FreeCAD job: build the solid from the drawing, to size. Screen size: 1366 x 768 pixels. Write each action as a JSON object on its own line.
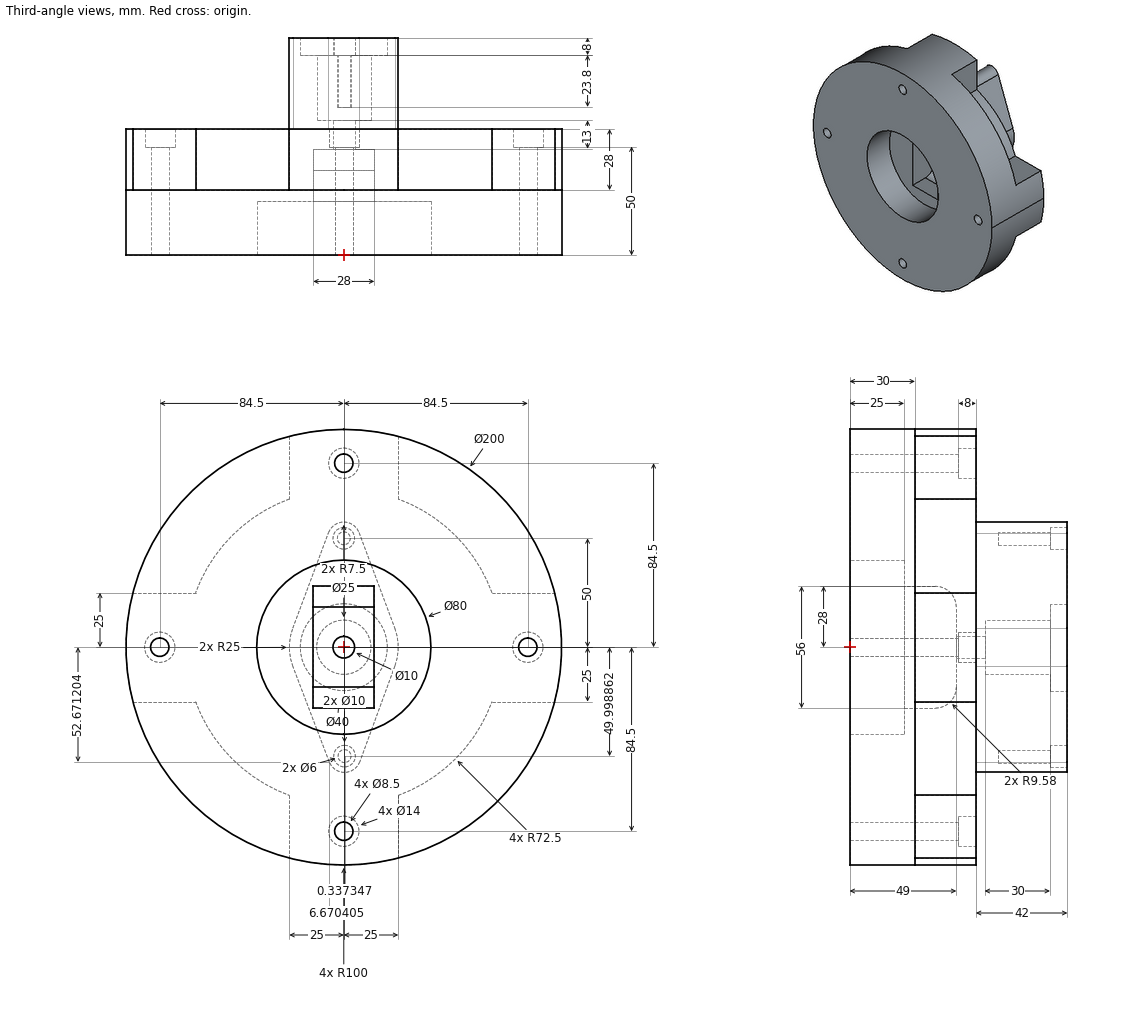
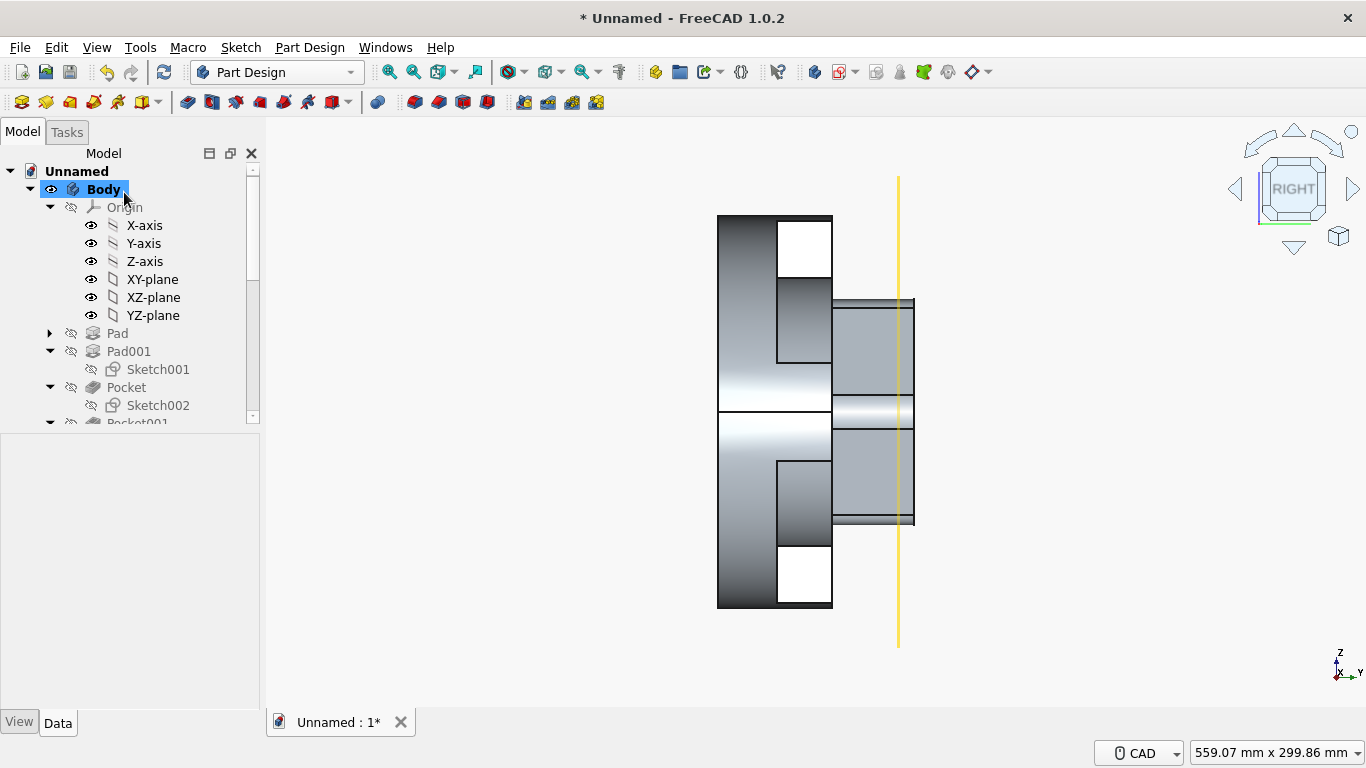
{"action": "scroll", "coordinate": [100, 293], "scroll_direction": "down", "scroll_amount": 3}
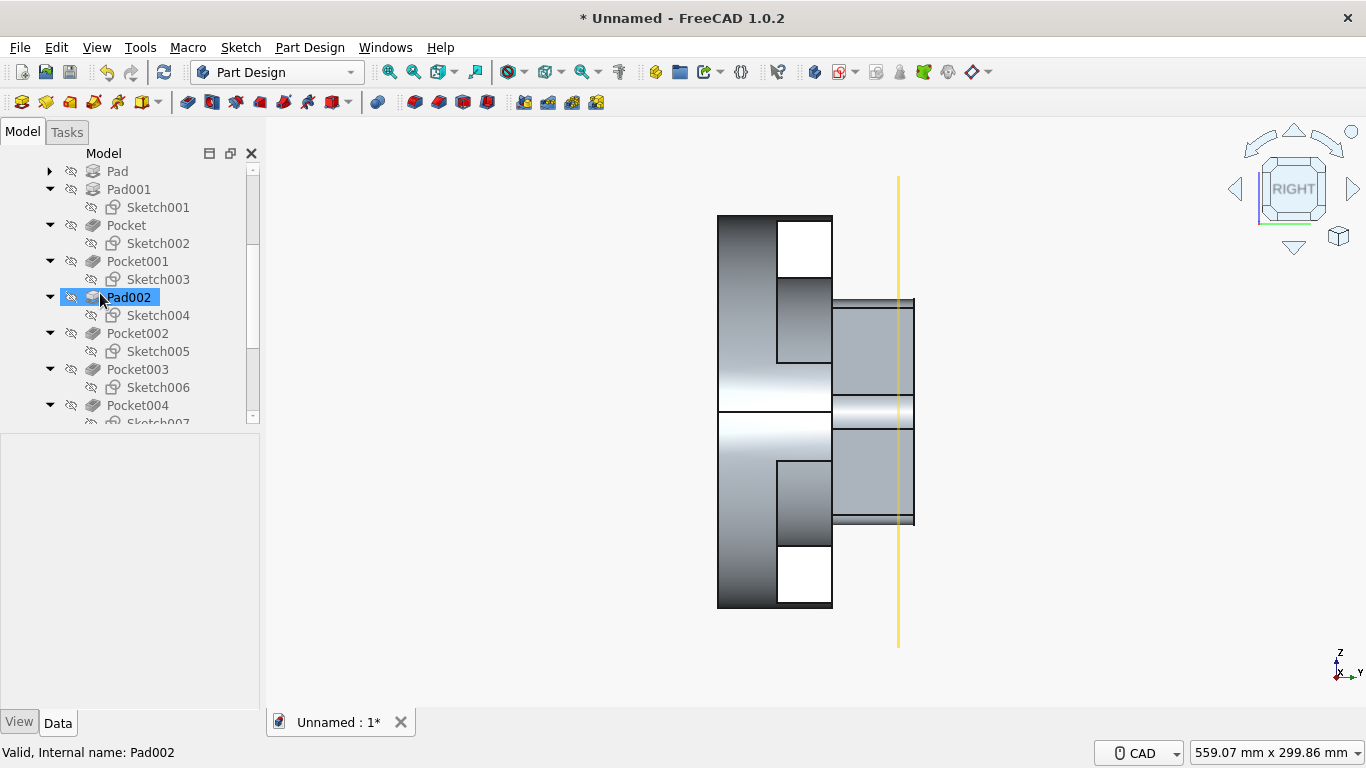
{"action": "scroll", "coordinate": [140, 293], "scroll_direction": "up", "scroll_amount": 15}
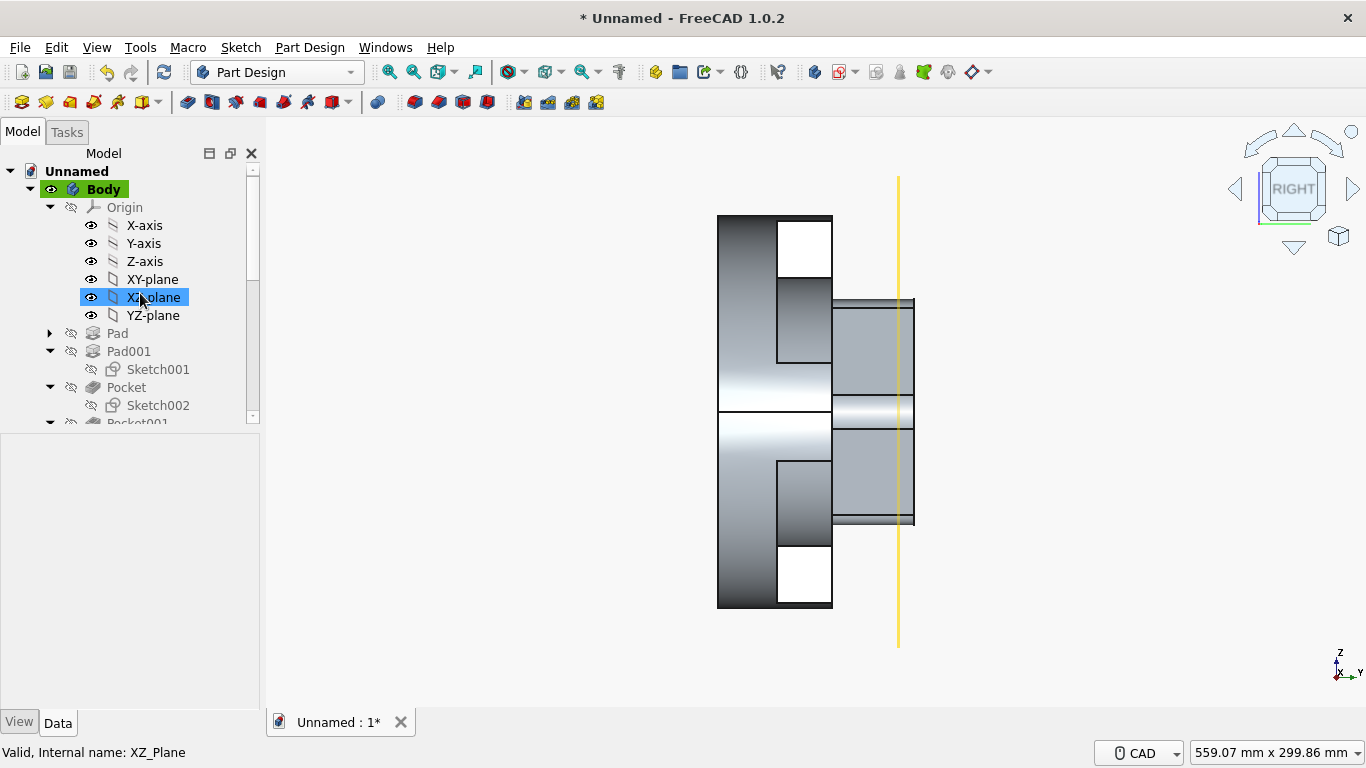
{"action": "scroll", "coordinate": [100, 293], "scroll_direction": "down", "scroll_amount": 6}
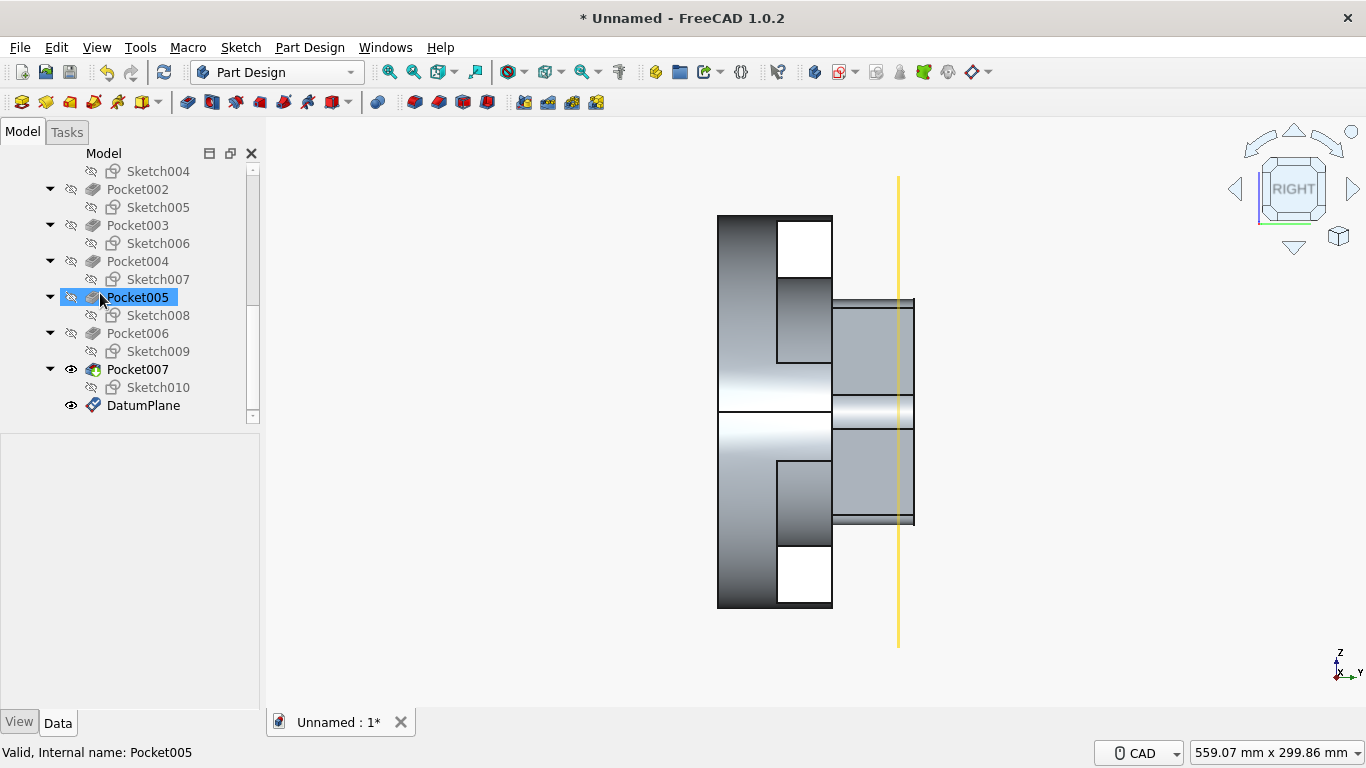
{"action": "left_click", "coordinate": [116, 405]}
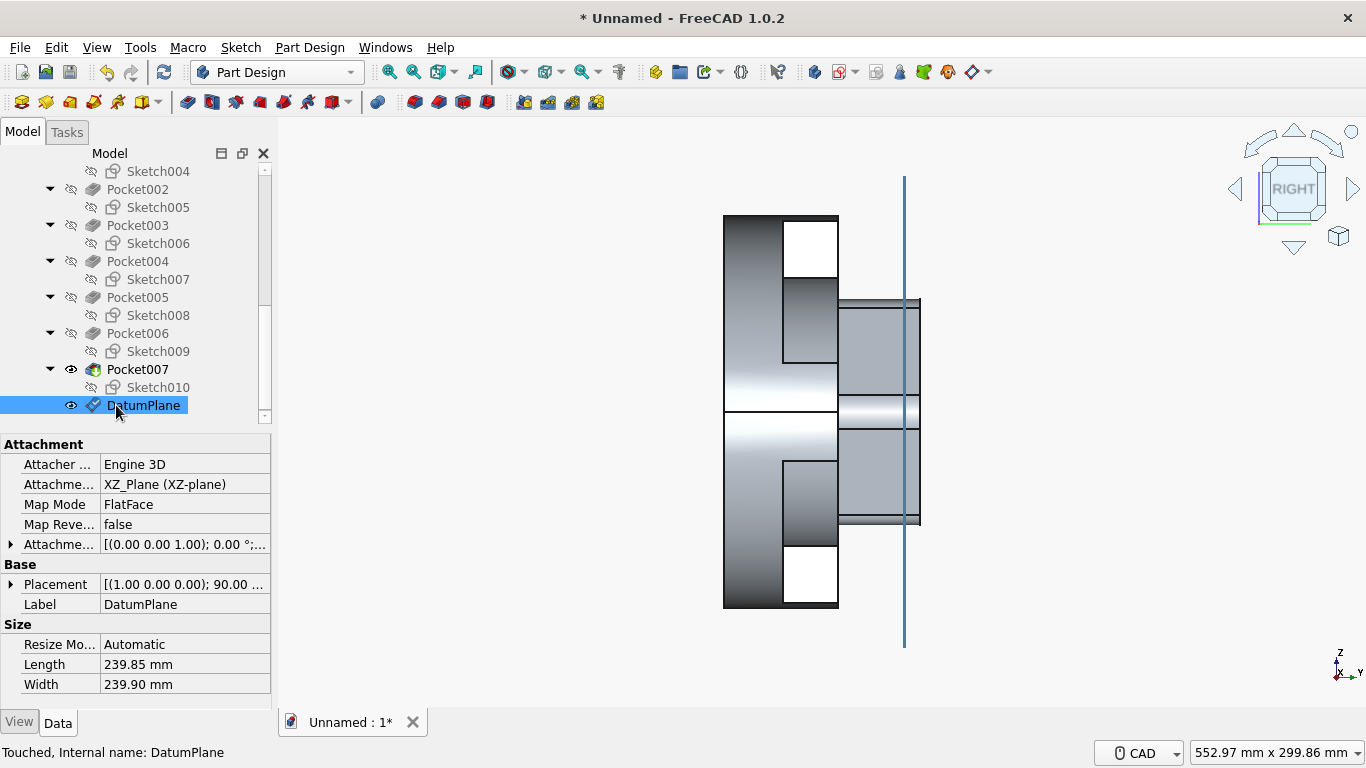
{"action": "left_click", "coordinate": [840, 72]}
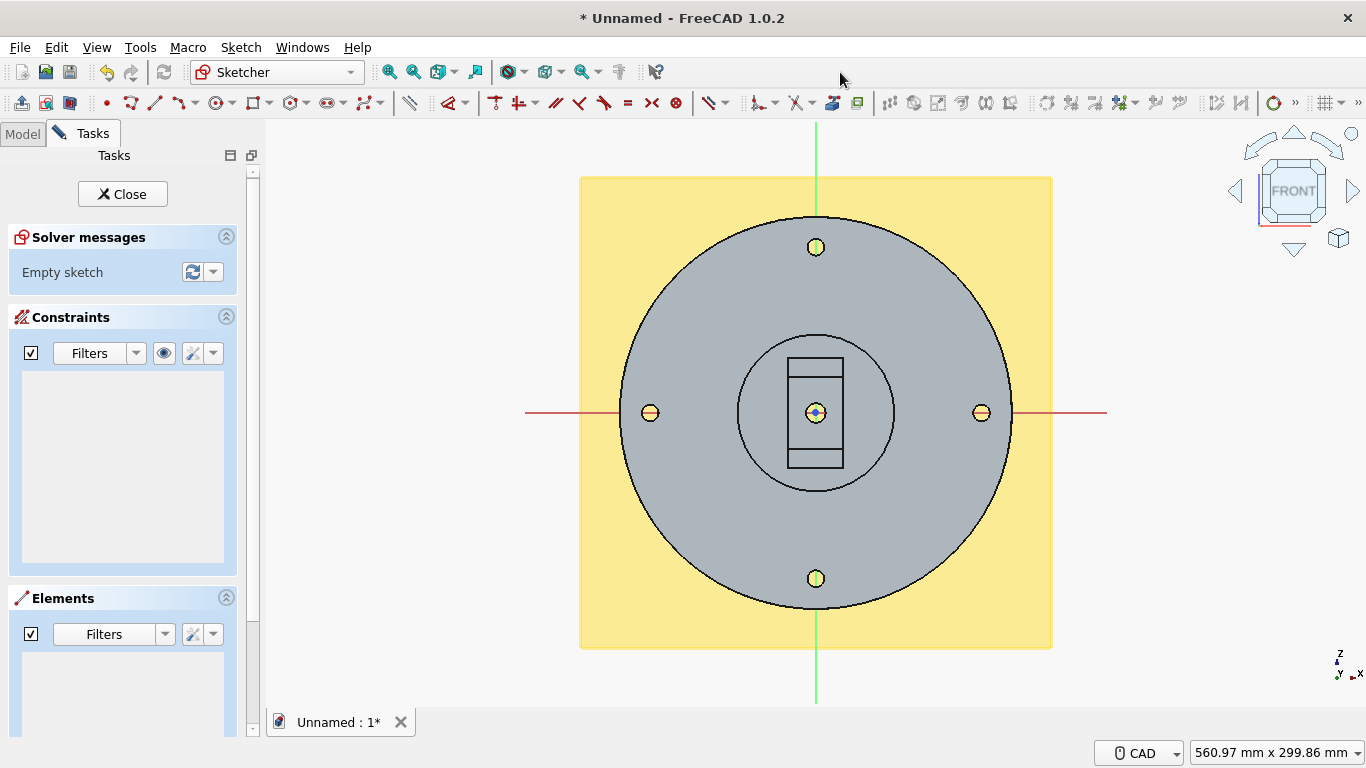
{"action": "key", "text": "q s"}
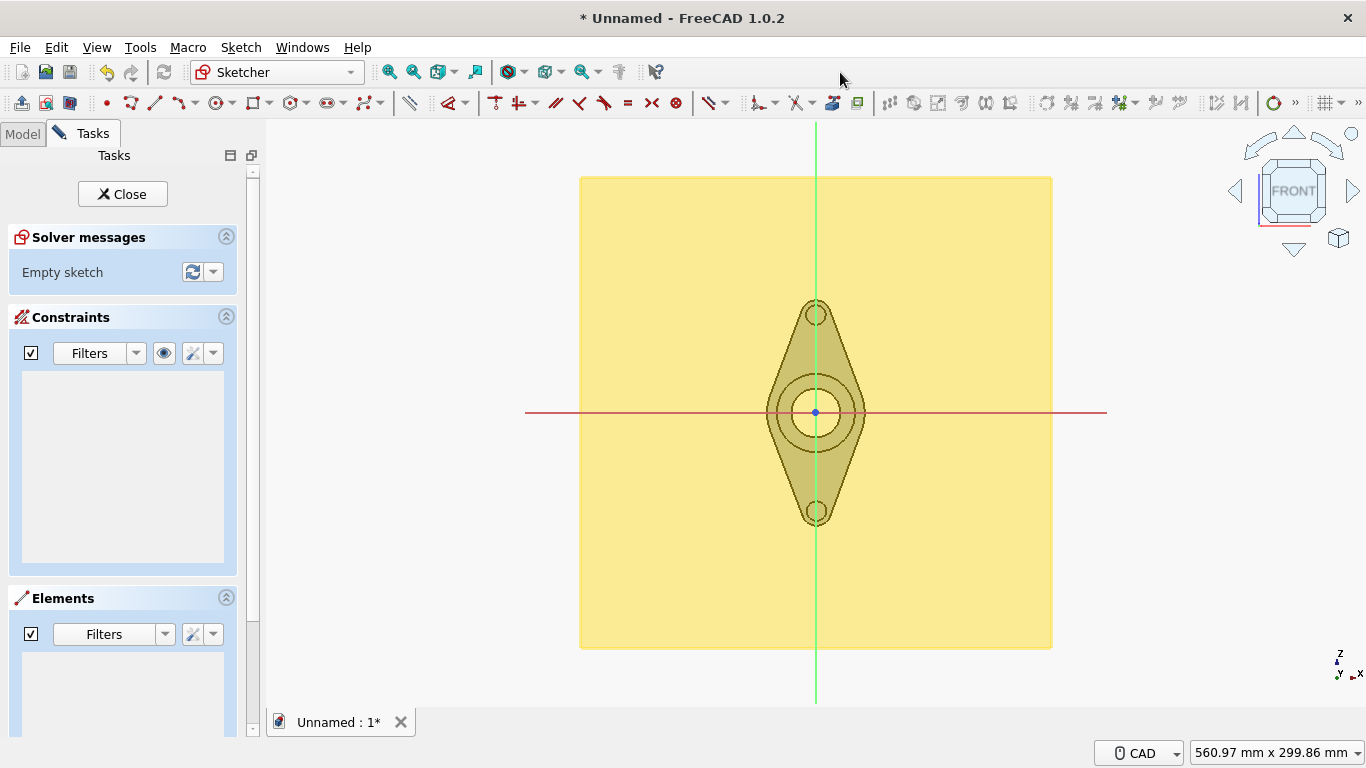
{"action": "scroll", "coordinate": [900, 413], "scroll_direction": "up", "scroll_amount": 3}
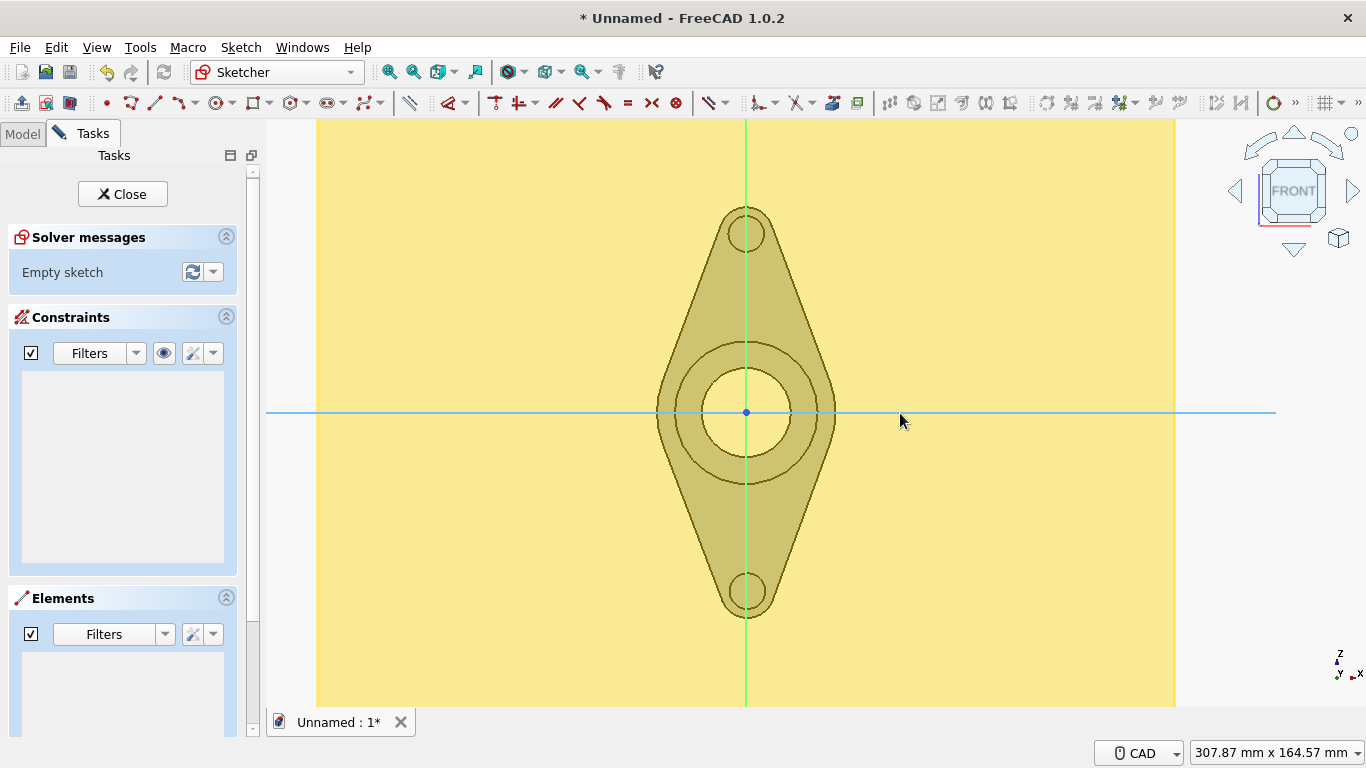
{"action": "left_click", "coordinate": [216, 104]}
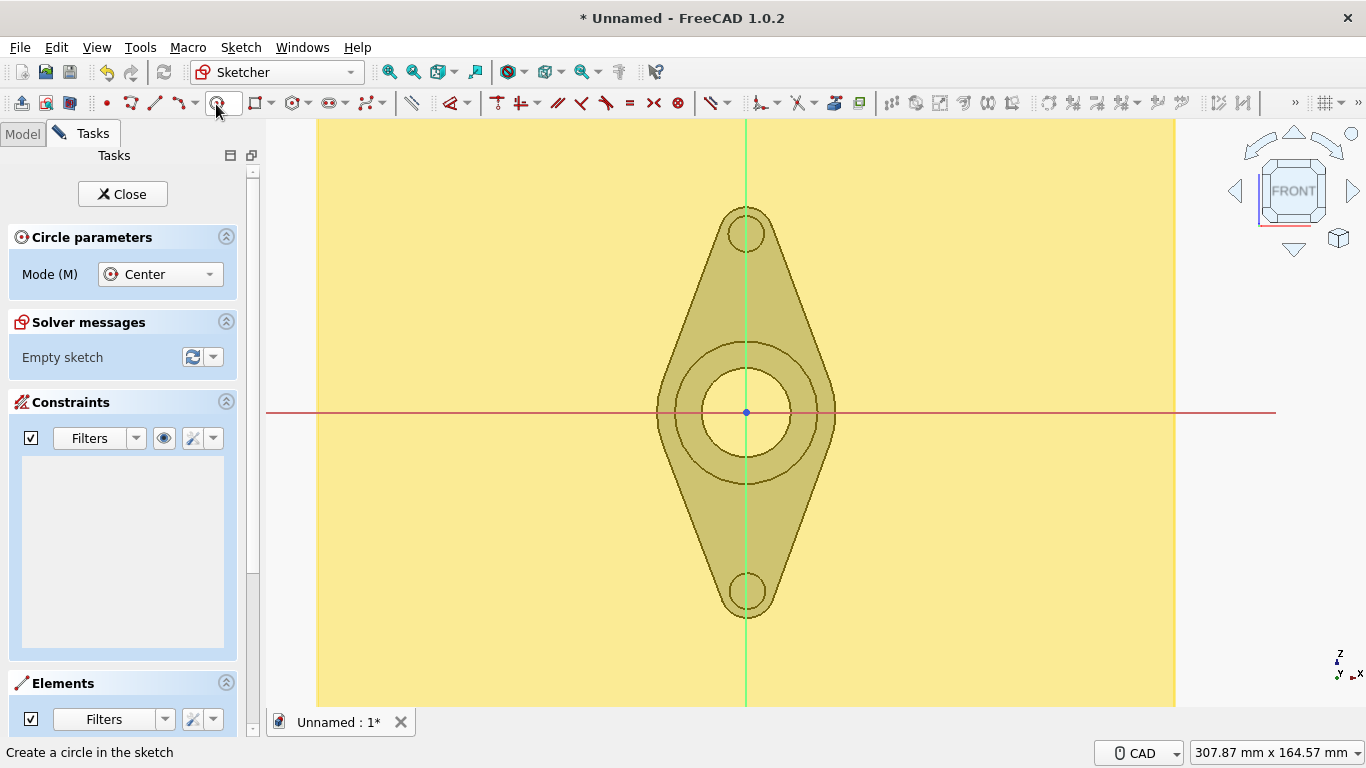
{"action": "scroll", "coordinate": [747, 591], "scroll_direction": "up", "scroll_amount": 13}